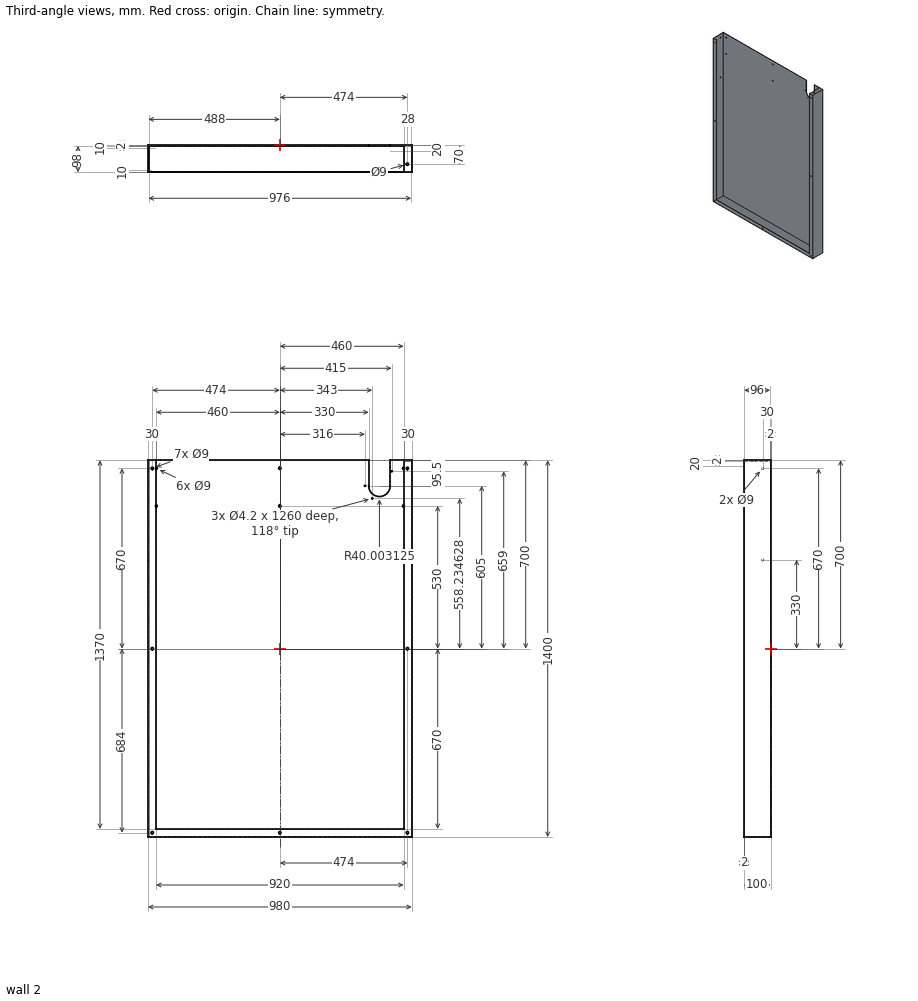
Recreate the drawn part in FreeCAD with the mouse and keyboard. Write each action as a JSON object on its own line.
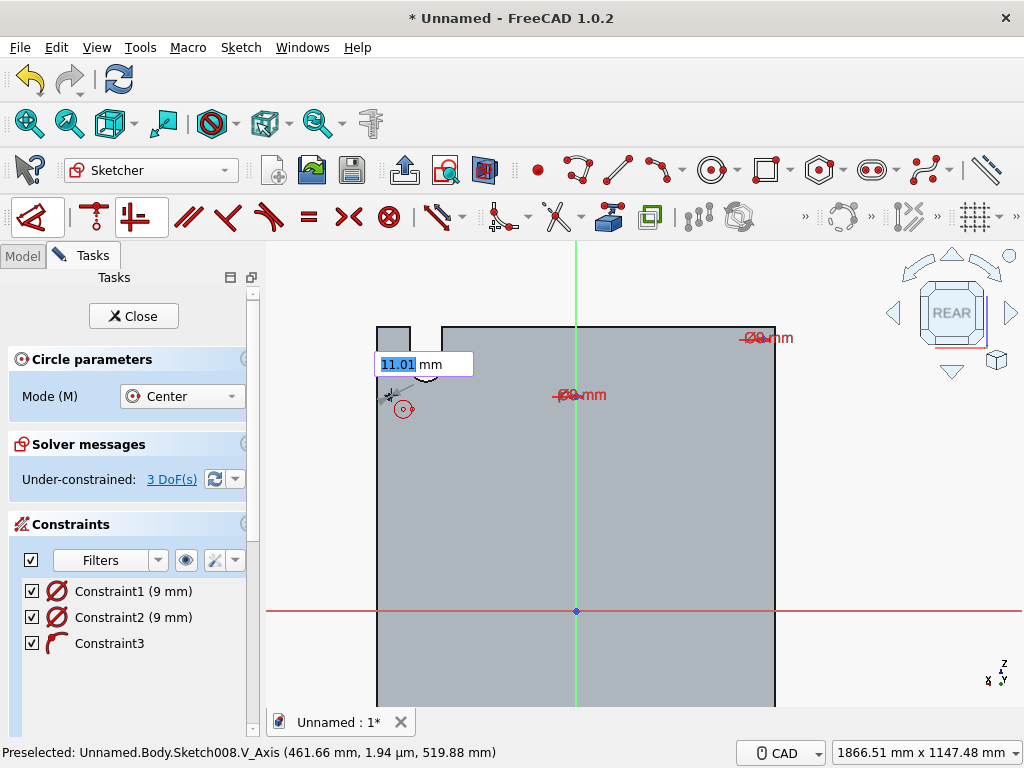
{"action": "type", "text": "9"}
{"action": "key", "text": "Return"}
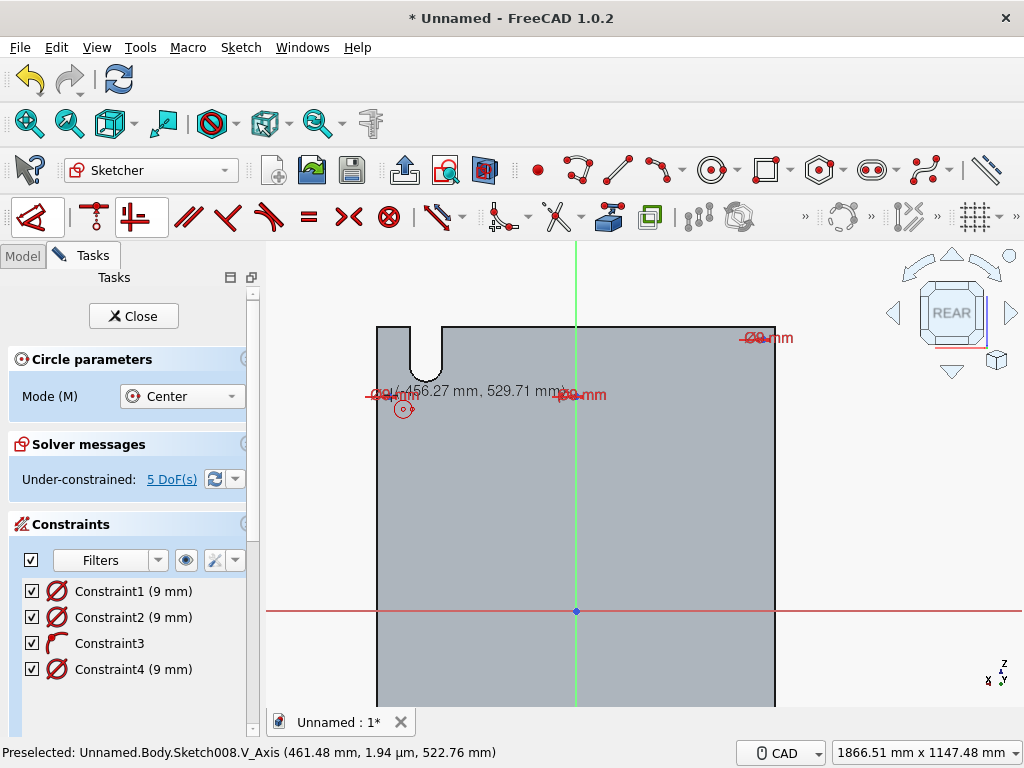
{"action": "scroll", "coordinate": [763, 396], "scroll_direction": "up", "scroll_amount": 13}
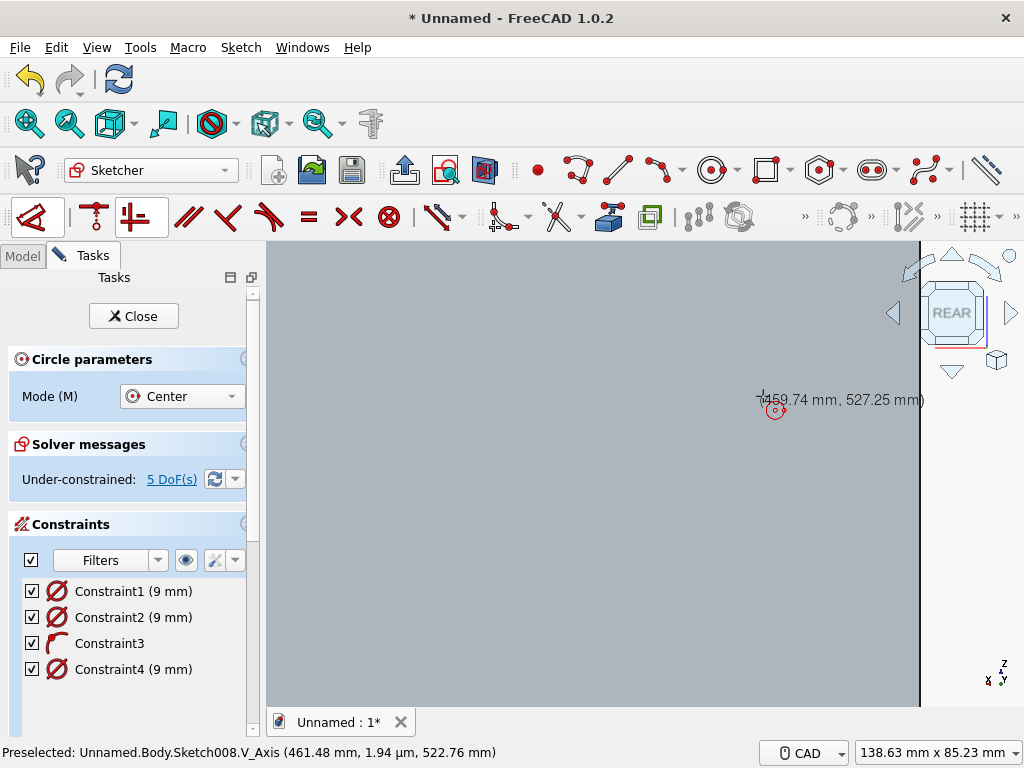
{"action": "scroll", "coordinate": [764, 396], "scroll_direction": "down", "scroll_amount": 13}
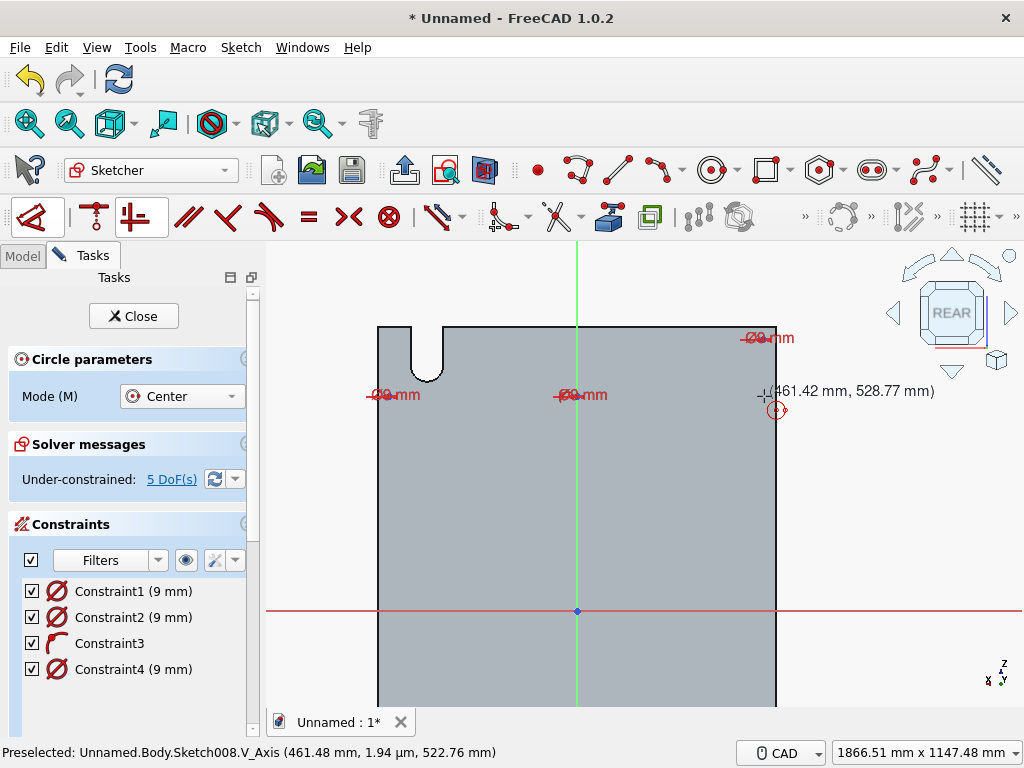
{"action": "left_click", "coordinate": [764, 396]}
{"action": "mouse_move", "coordinate": [765, 395]}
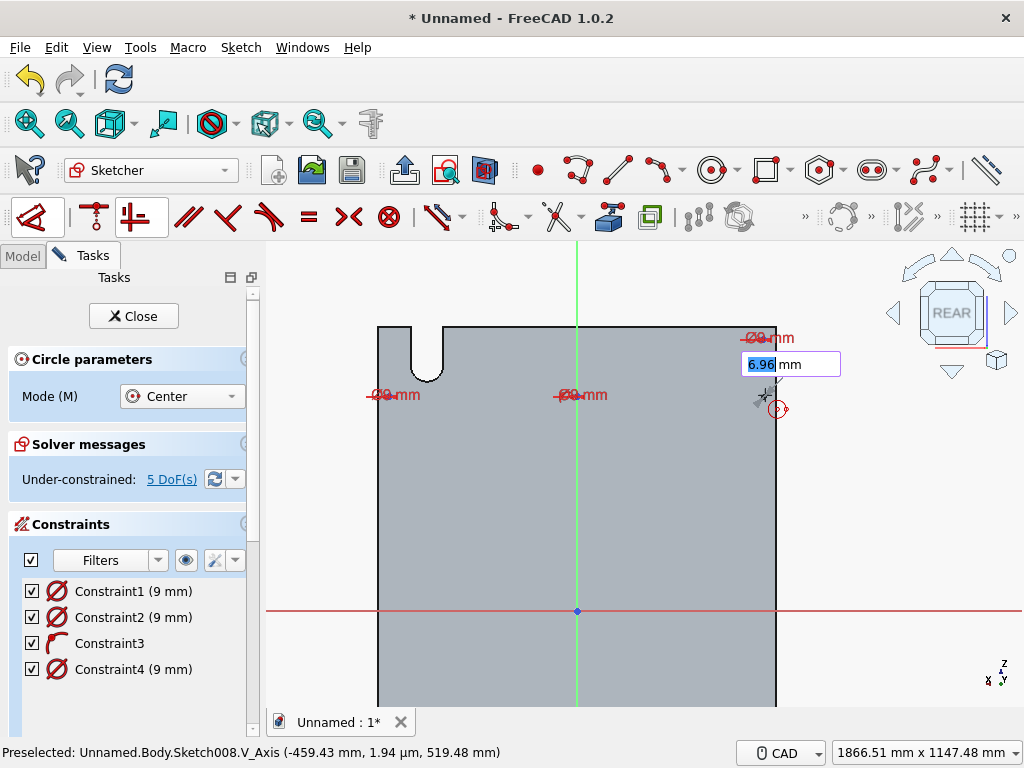
{"action": "type", "text": "9"}
{"action": "key", "text": "Return"}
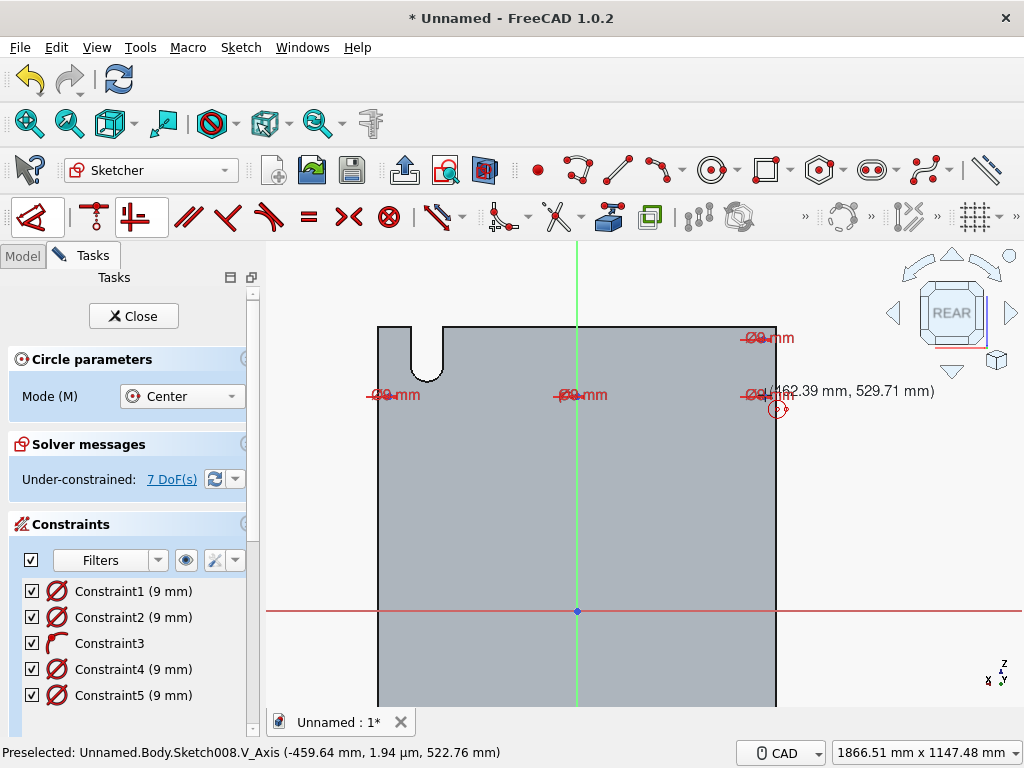
{"action": "scroll", "coordinate": [577, 339], "scroll_direction": "up", "scroll_amount": 13}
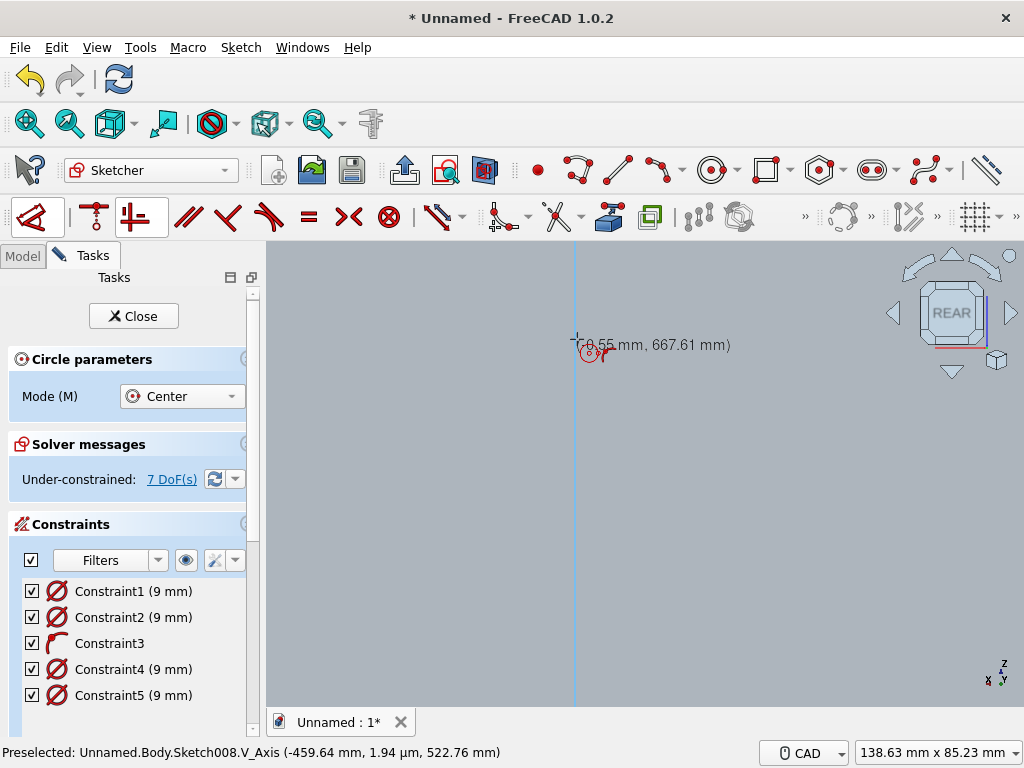
{"action": "scroll", "coordinate": [577, 339], "scroll_direction": "down", "scroll_amount": 13}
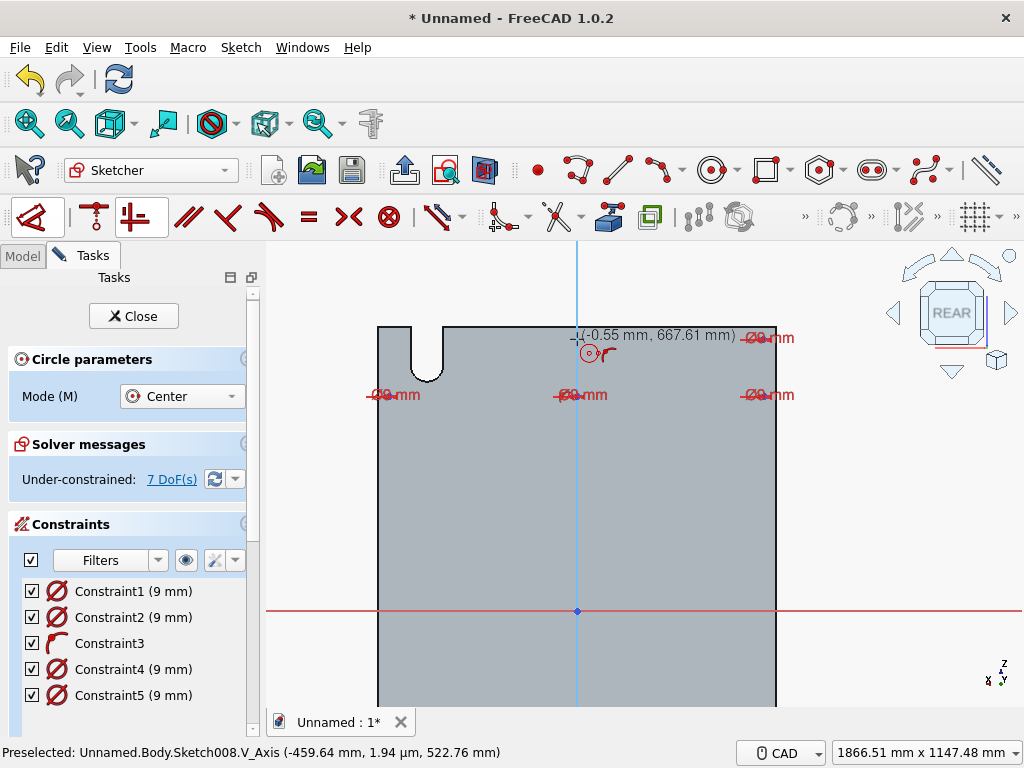
{"action": "left_click", "coordinate": [577, 339]}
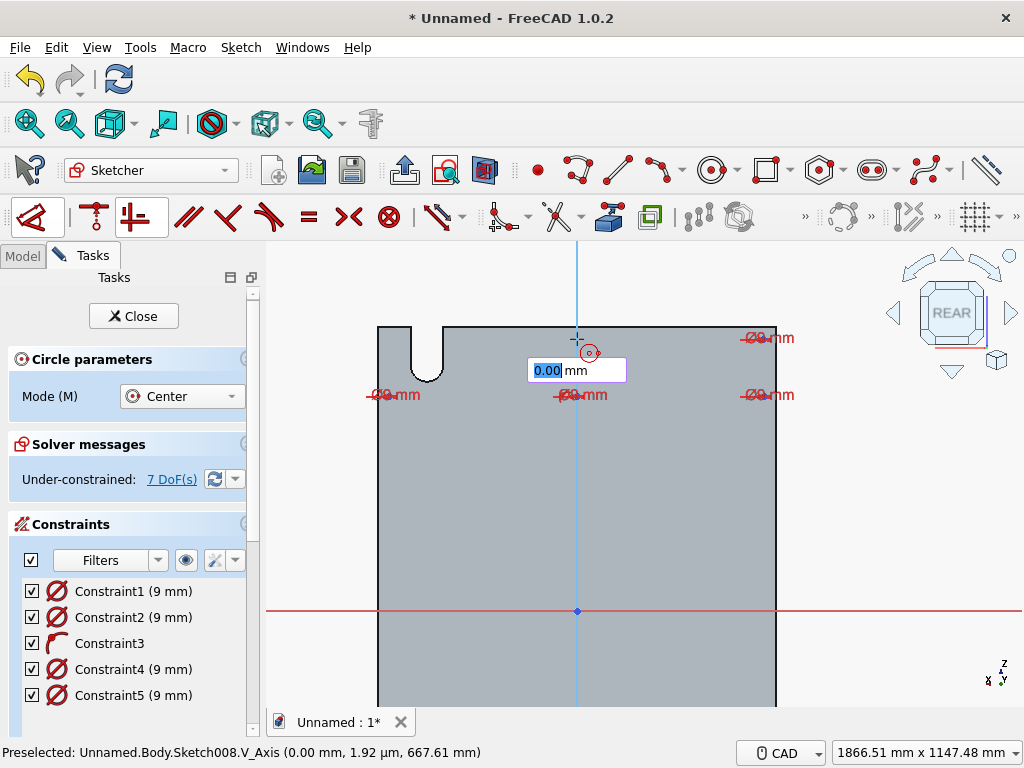
{"action": "scroll", "coordinate": [579, 338], "scroll_direction": "up", "scroll_amount": 12}
{"action": "mouse_move", "coordinate": [574, 340]}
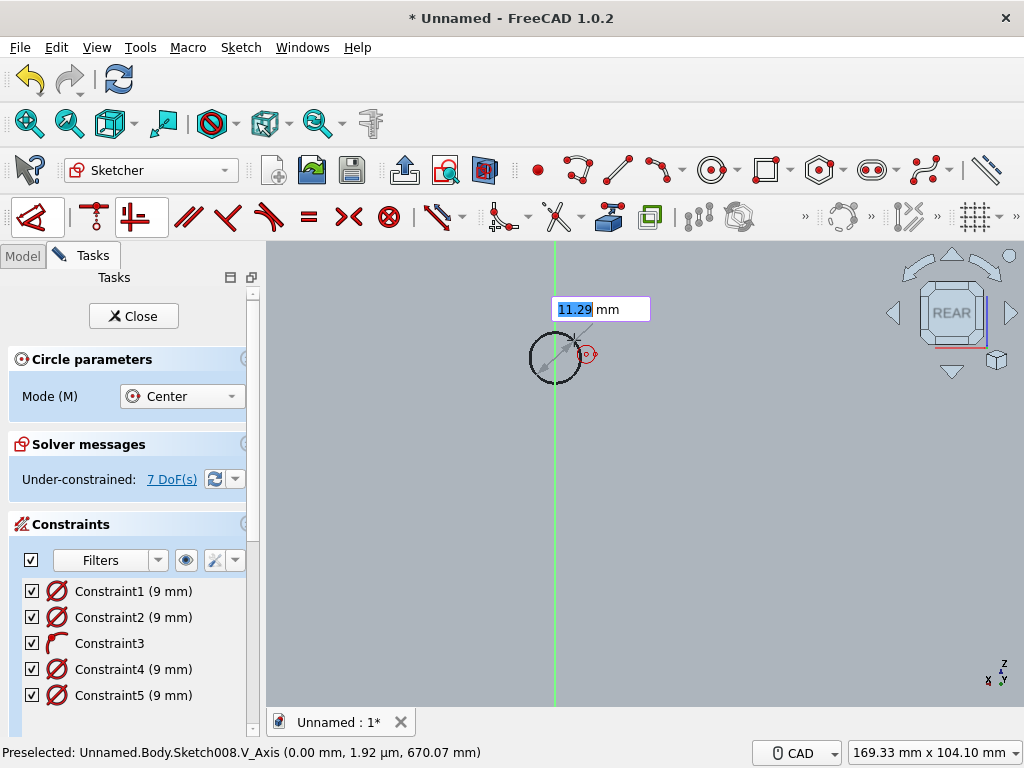
{"action": "type", "text": "9"}
{"action": "key", "text": "Return"}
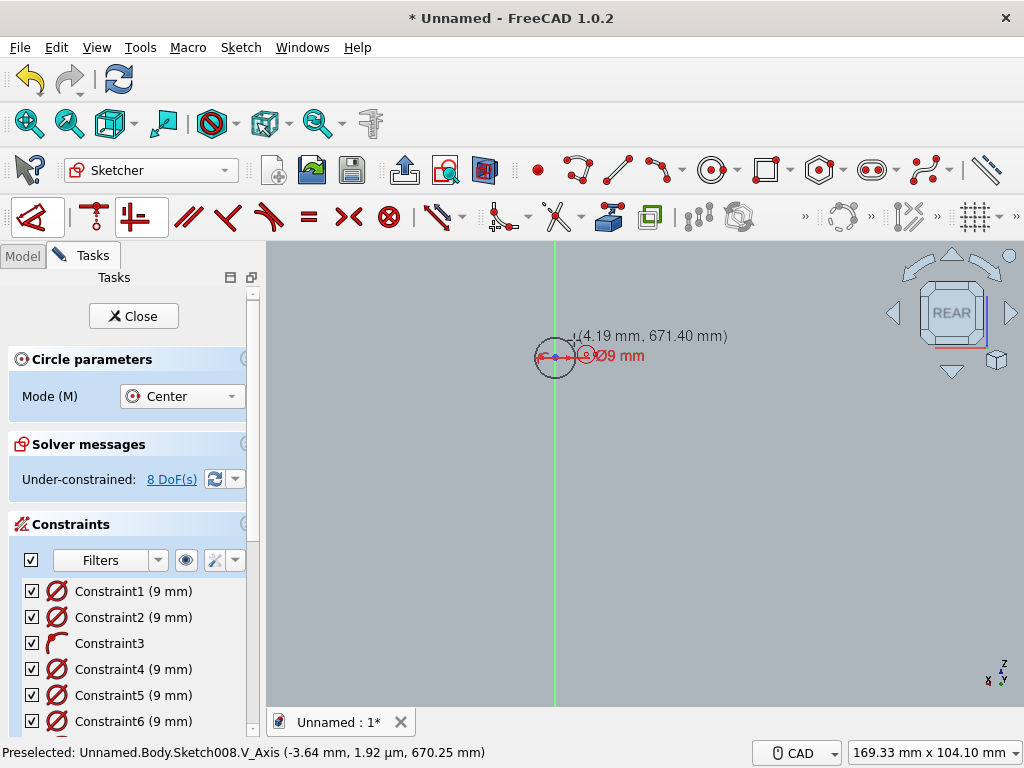
{"action": "scroll", "coordinate": [579, 338], "scroll_direction": "down", "scroll_amount": 12}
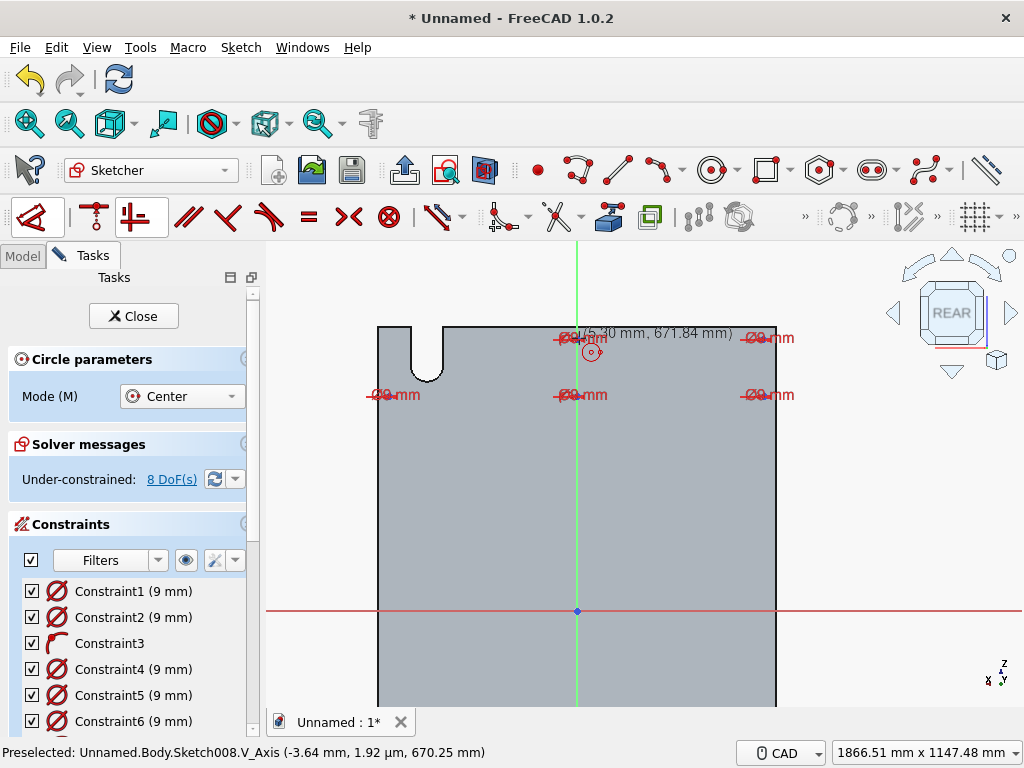
{"action": "scroll", "coordinate": [390, 339], "scroll_direction": "up", "scroll_amount": 13}